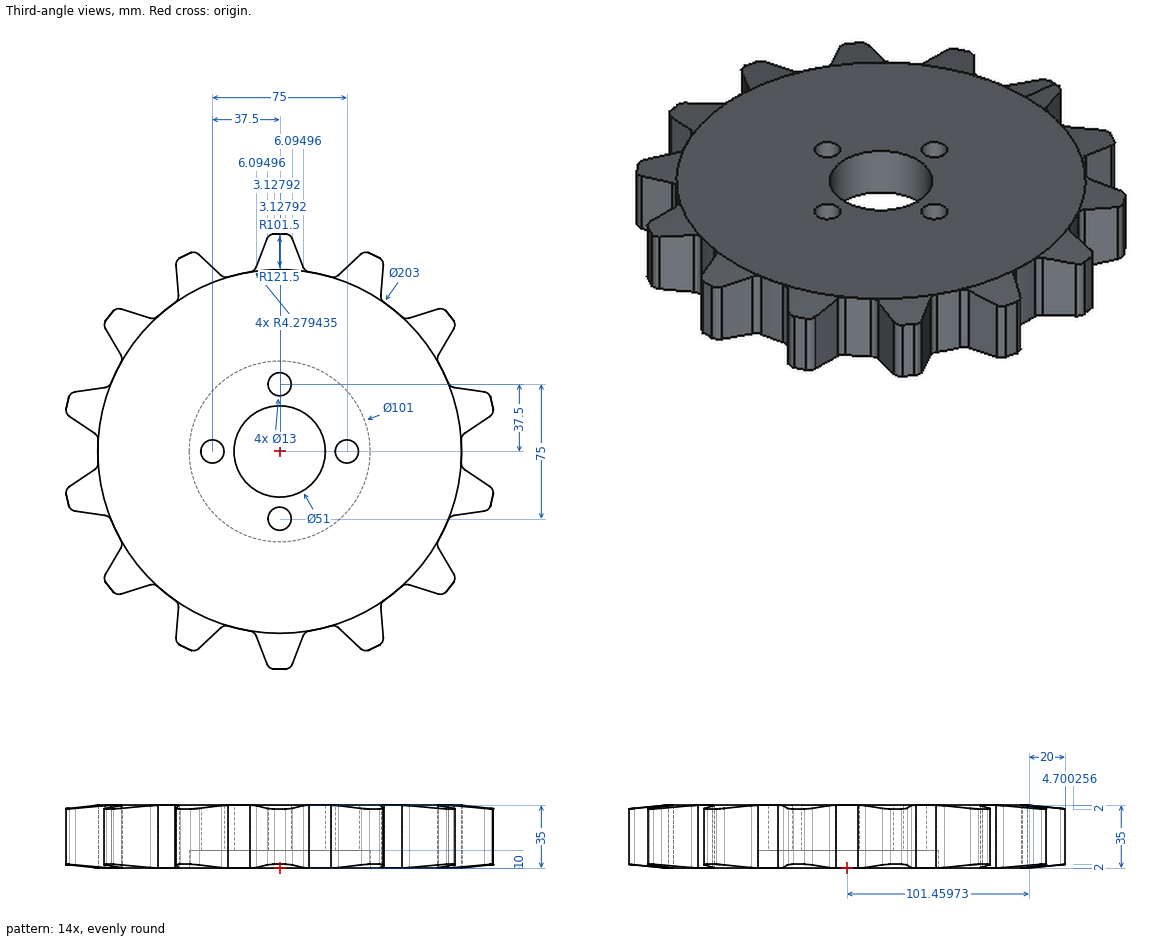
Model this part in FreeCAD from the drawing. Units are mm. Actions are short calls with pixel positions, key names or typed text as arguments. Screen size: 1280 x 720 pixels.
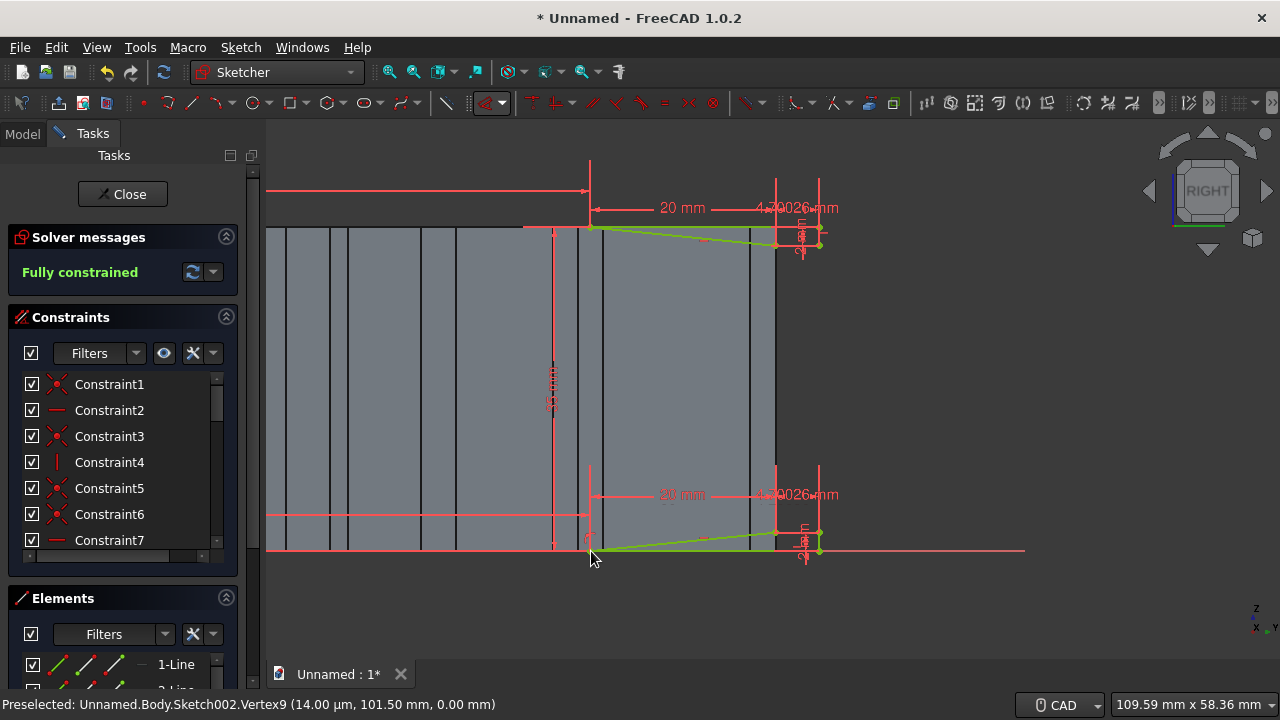
click(123, 194)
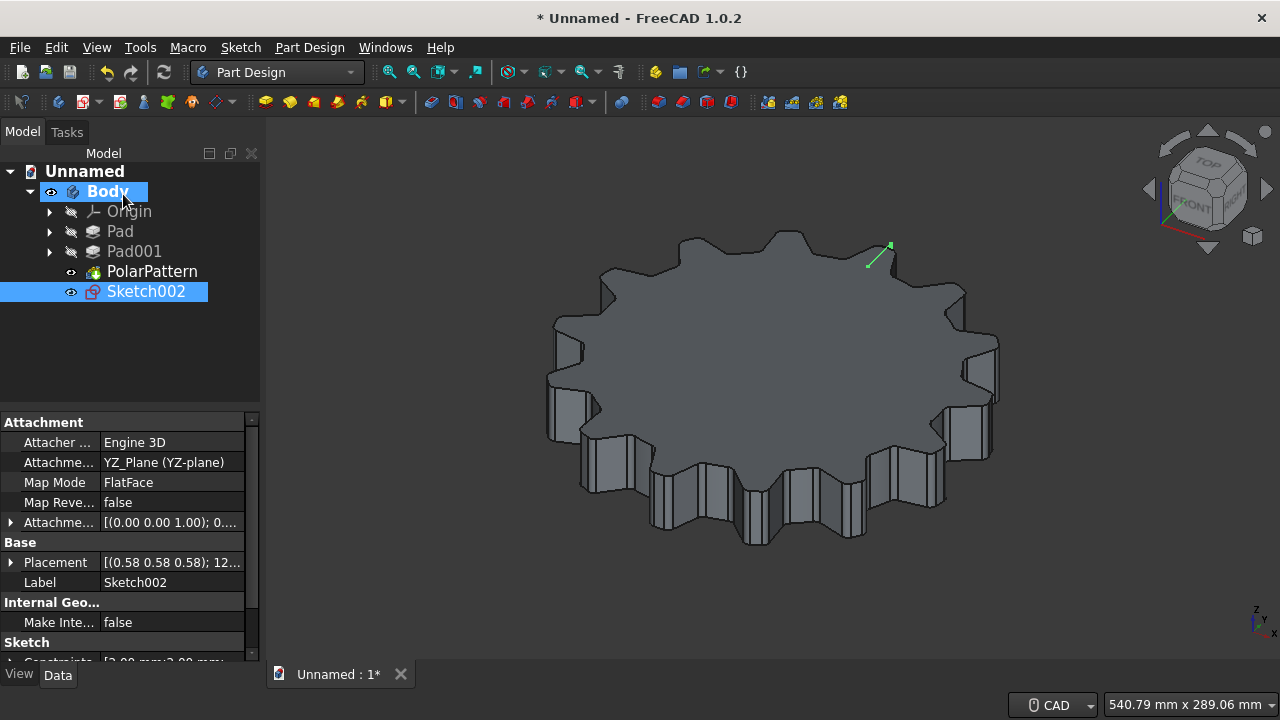
click(480, 102)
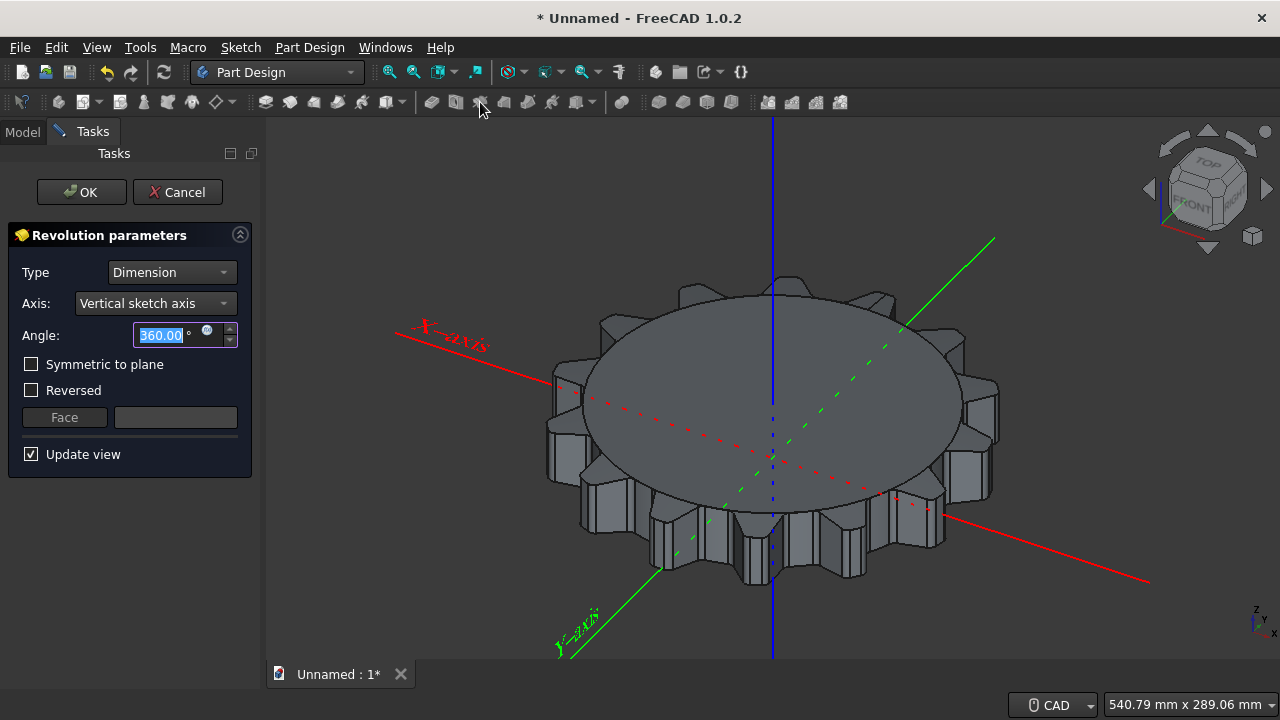
click(82, 192)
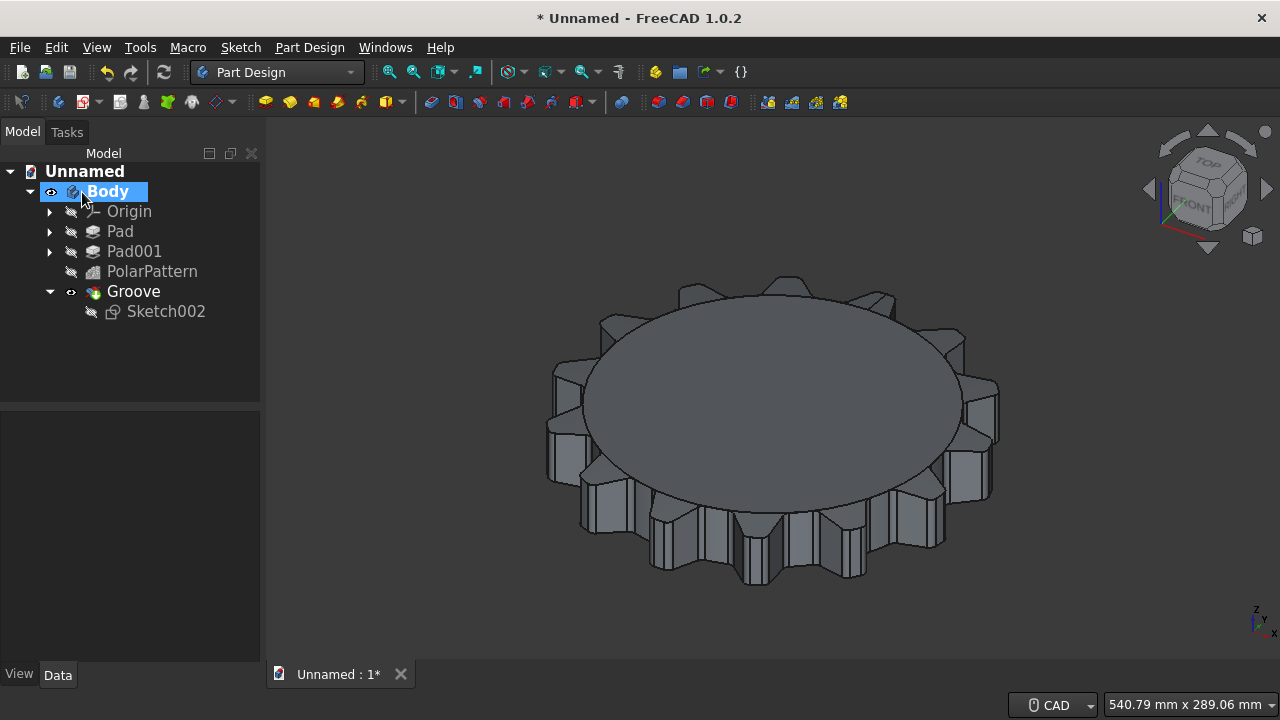
click(773, 403)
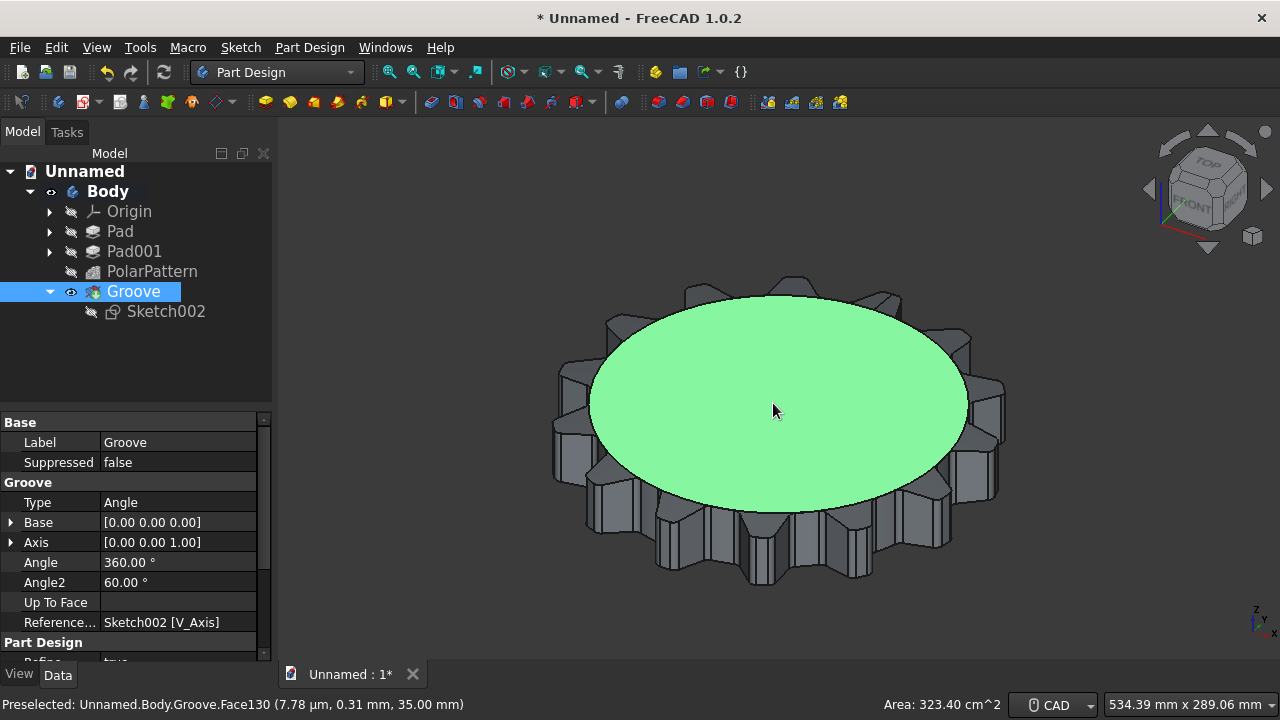
click(84, 102)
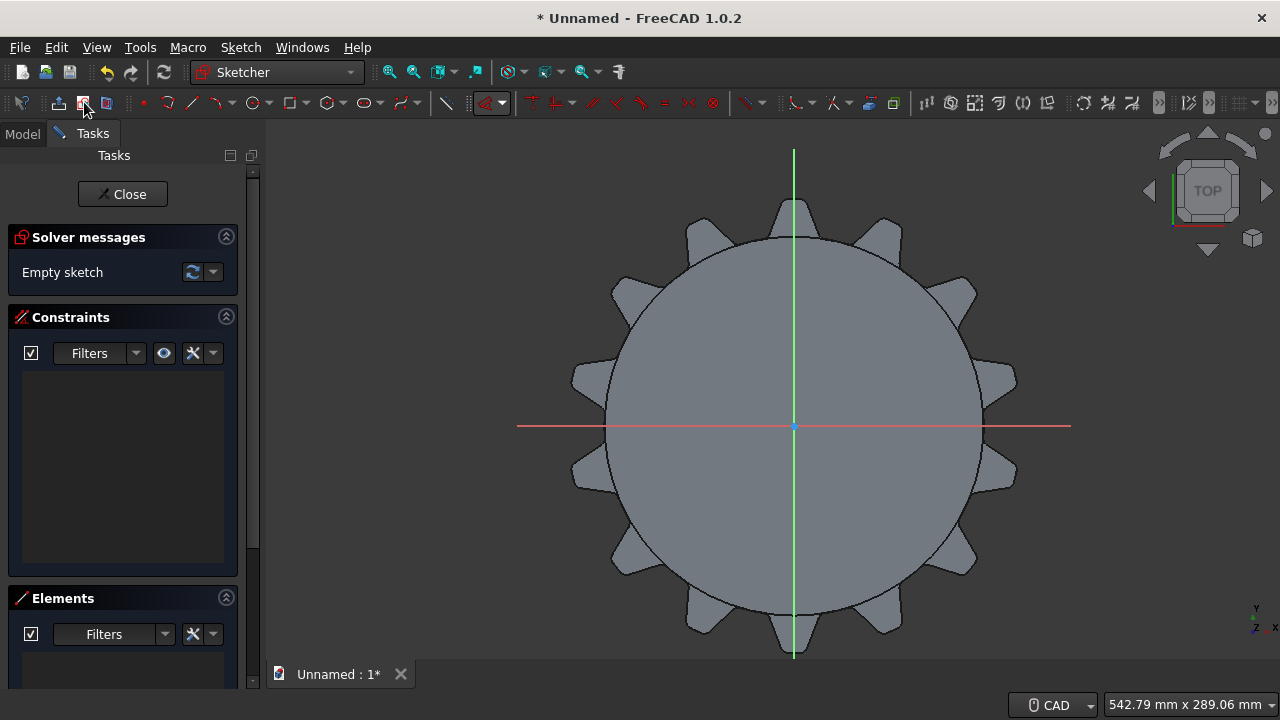
scroll(833, 442, up, 6)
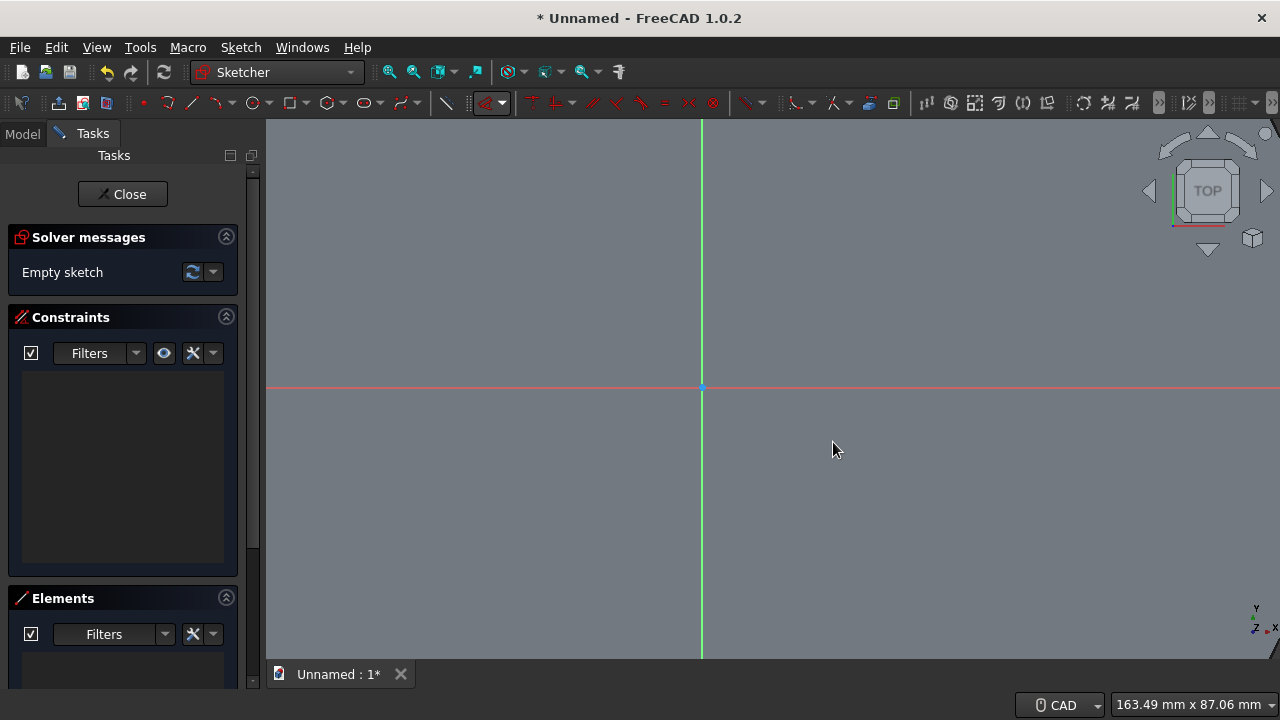
click(254, 104)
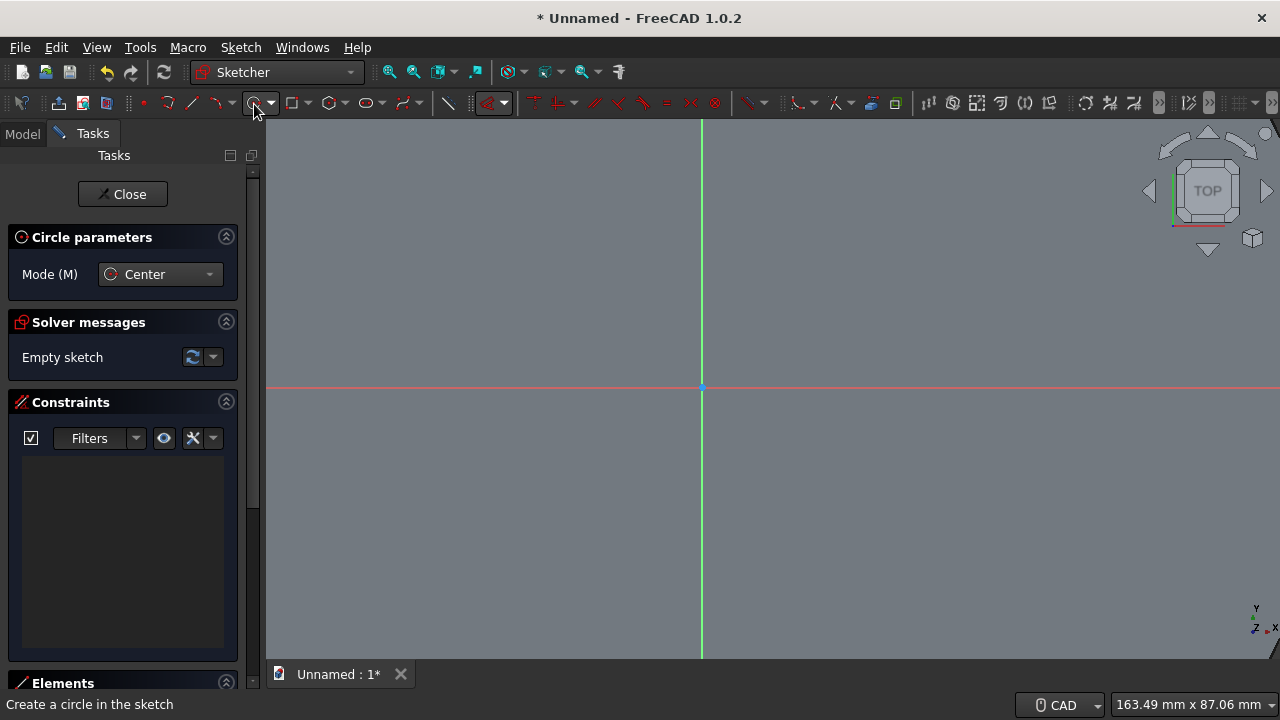
click(702, 388)
move(814, 276)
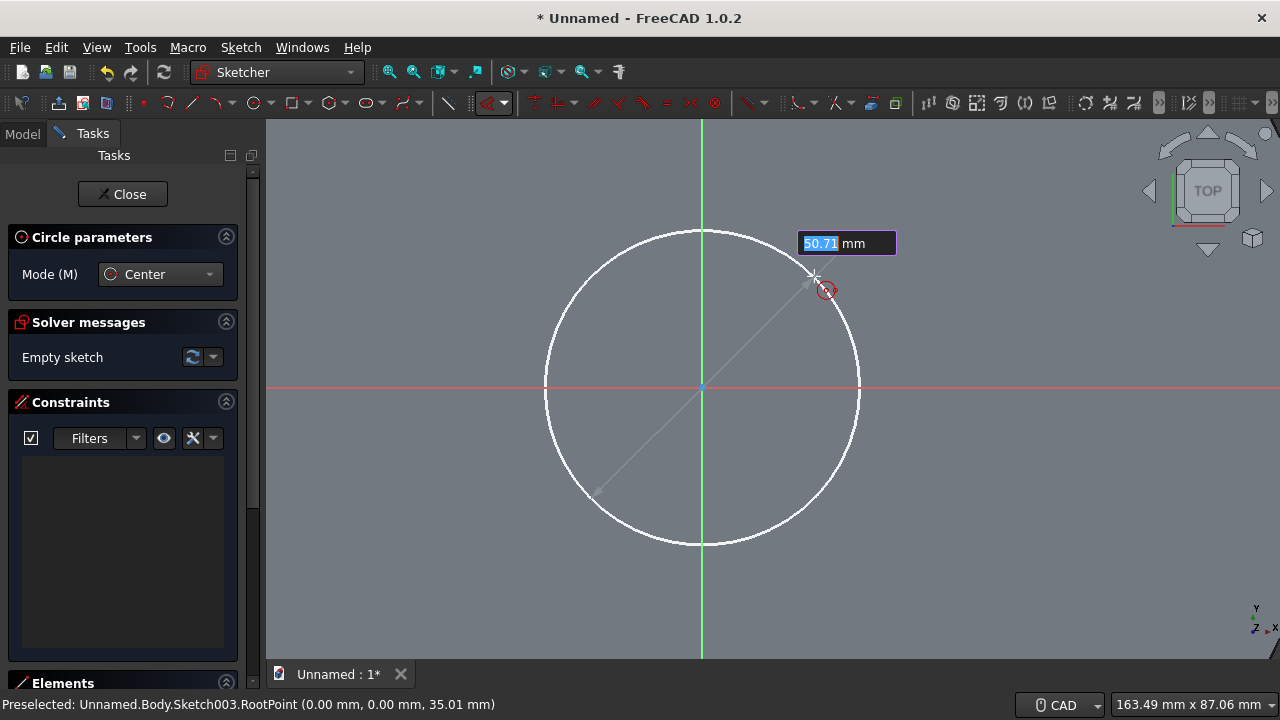
text(51)
key(Return)
key(Escape)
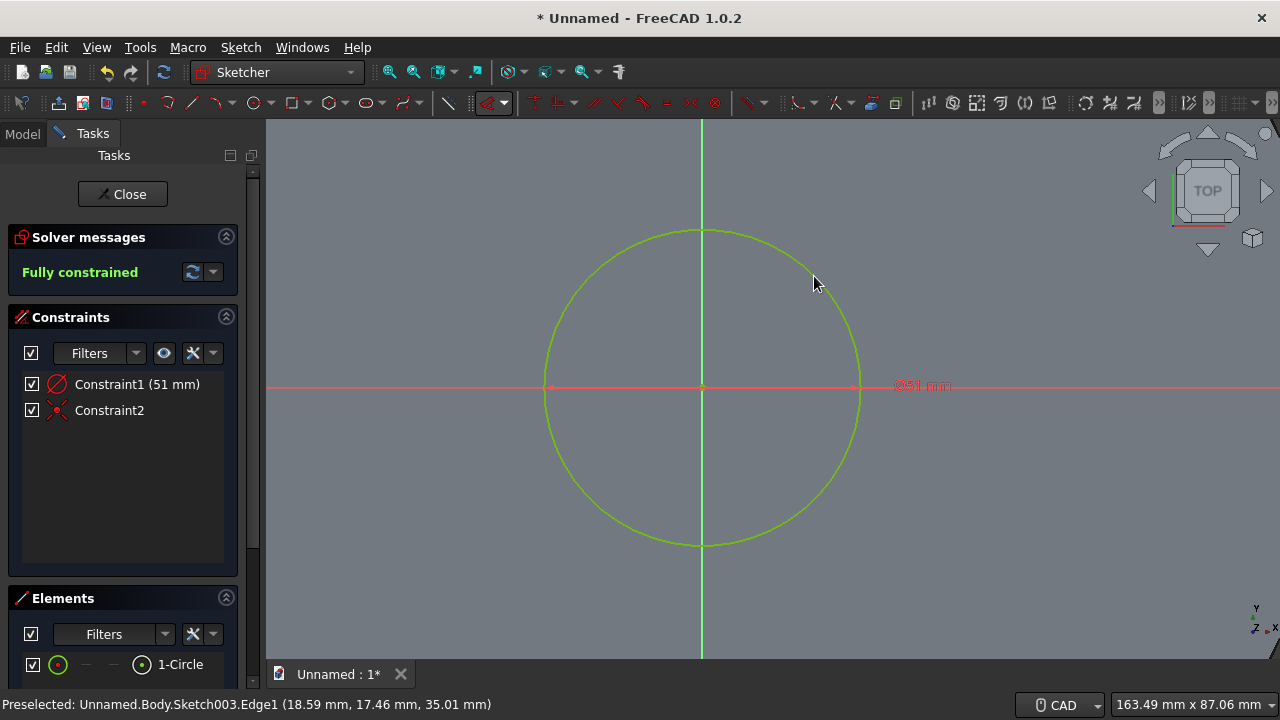
click(123, 194)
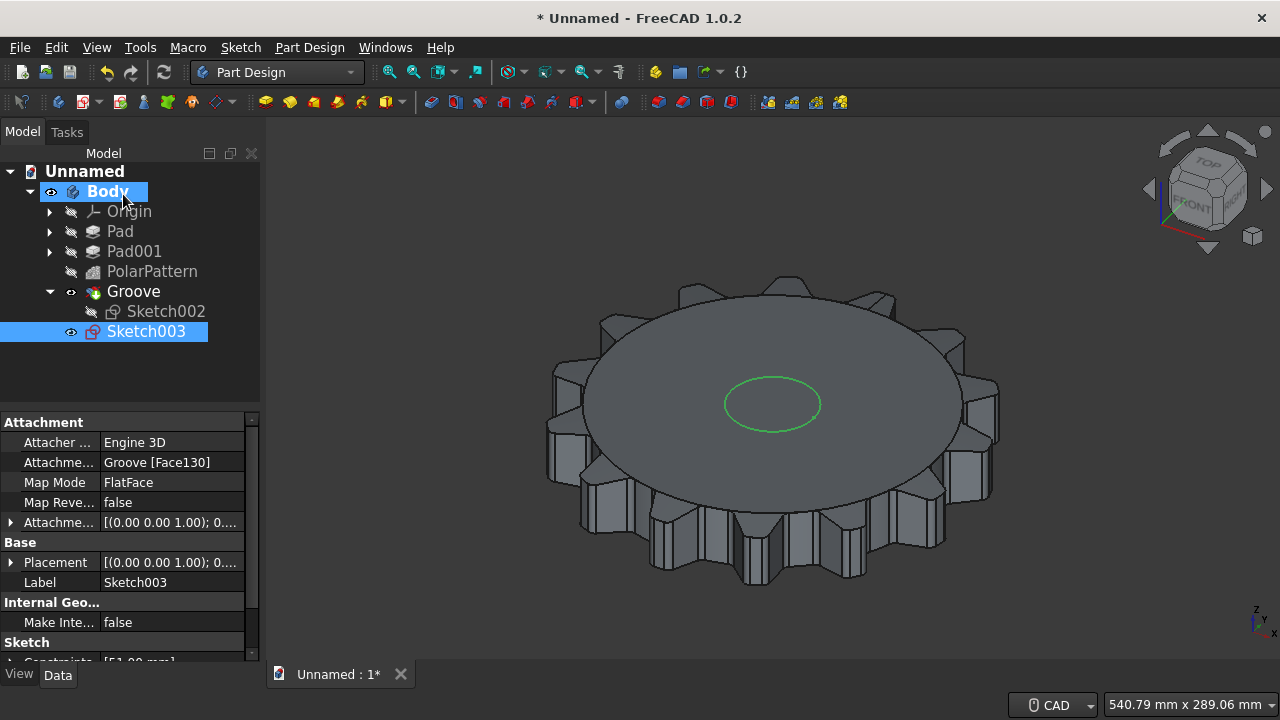
click(432, 102)